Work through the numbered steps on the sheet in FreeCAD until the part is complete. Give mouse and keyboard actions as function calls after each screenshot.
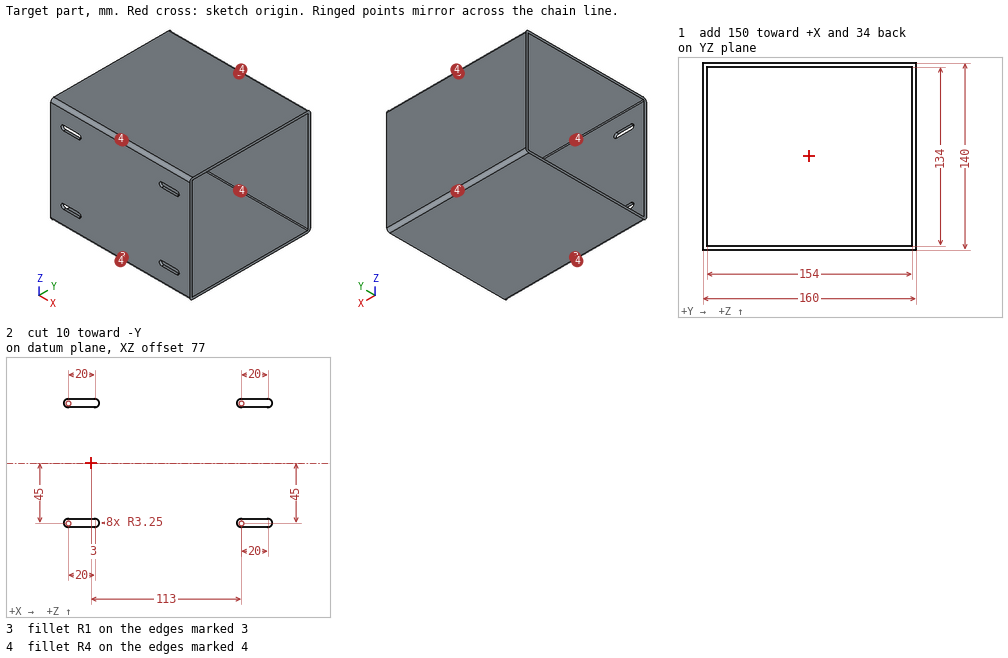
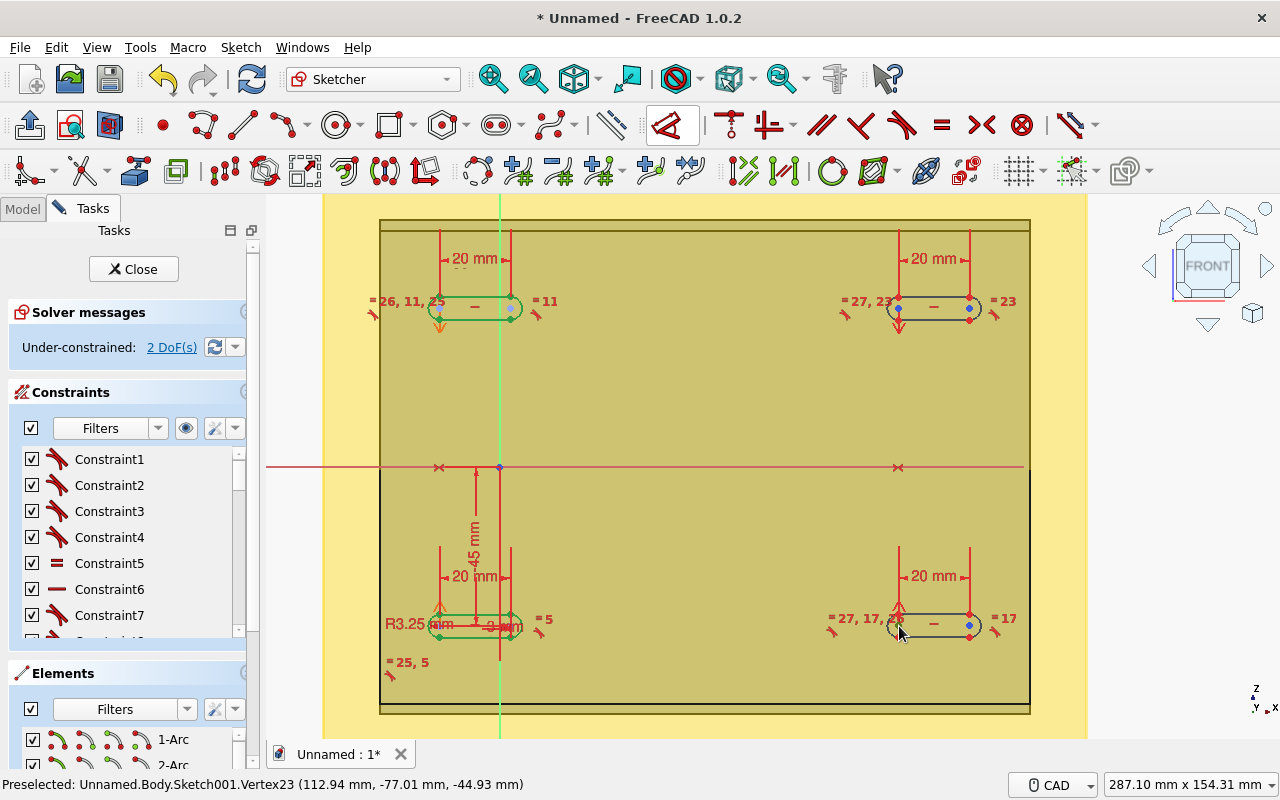
key(i)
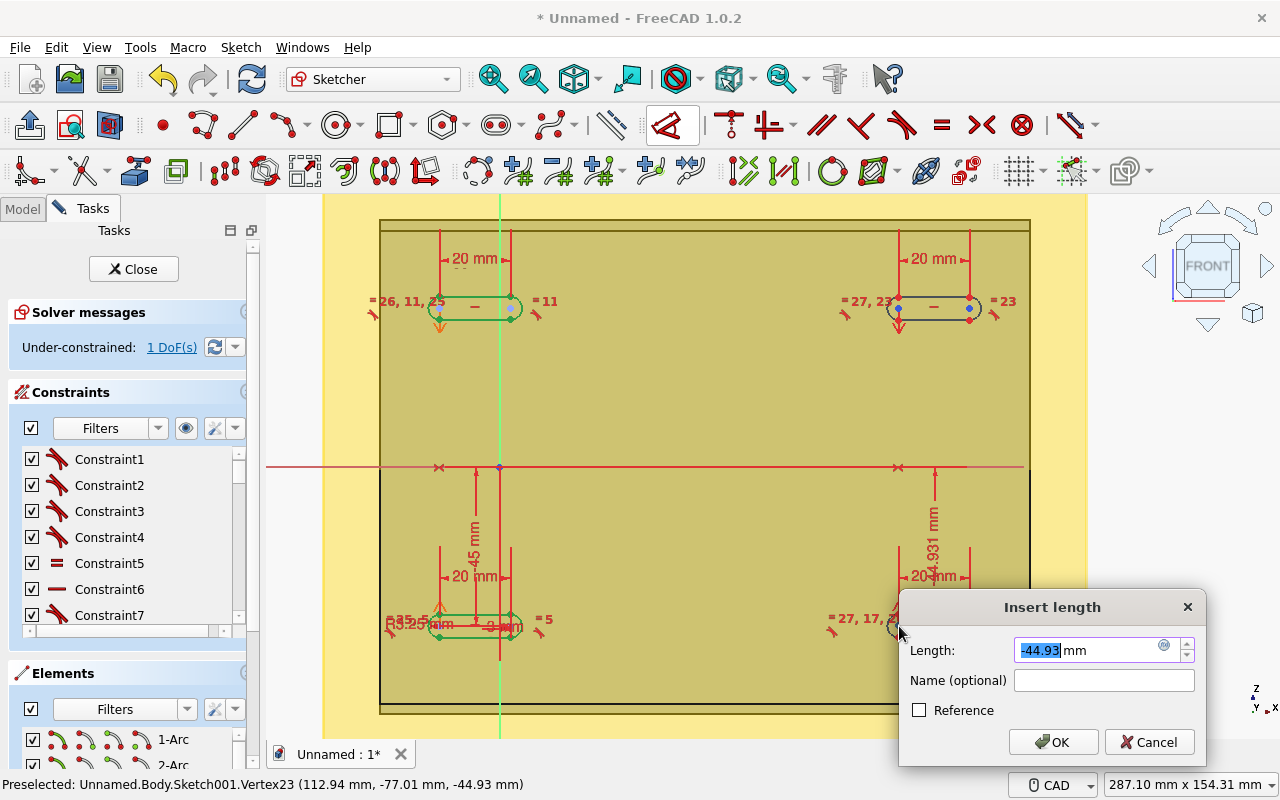
text(-45)
key(Return)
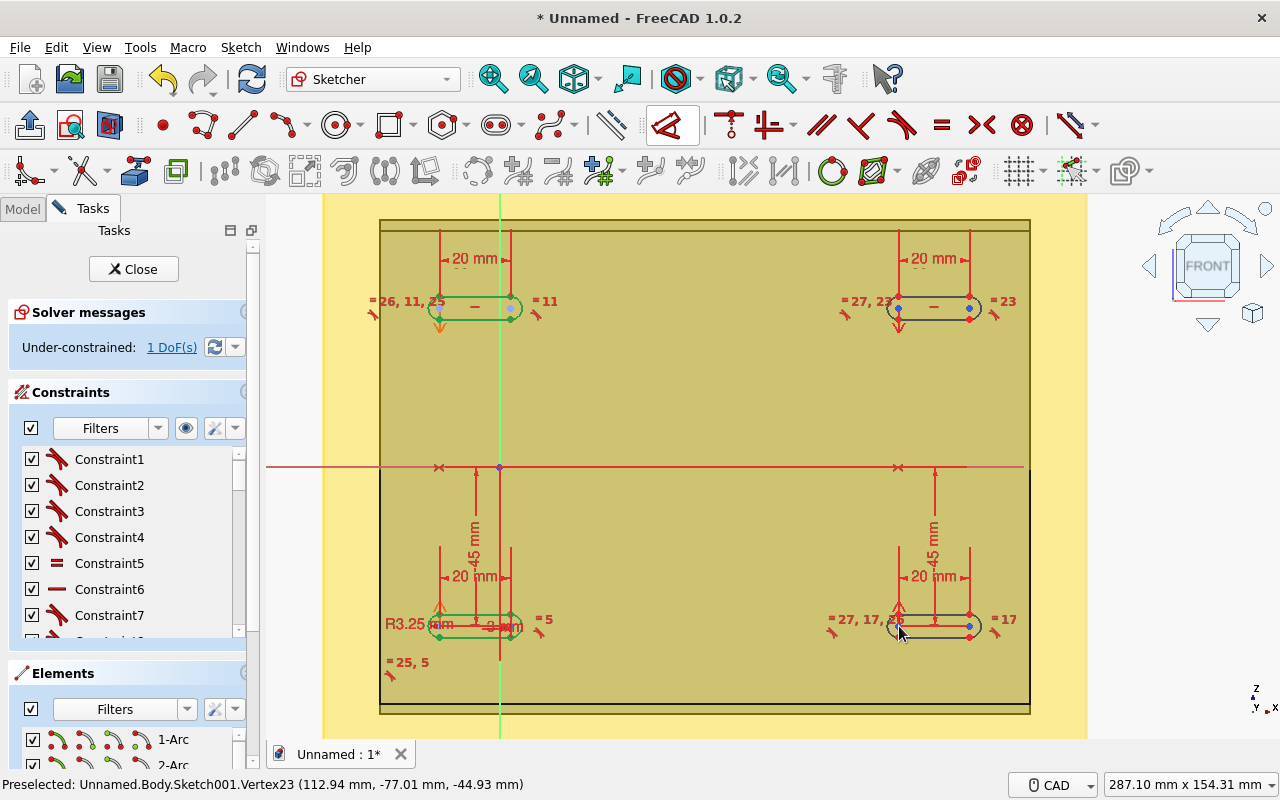
click(899, 615)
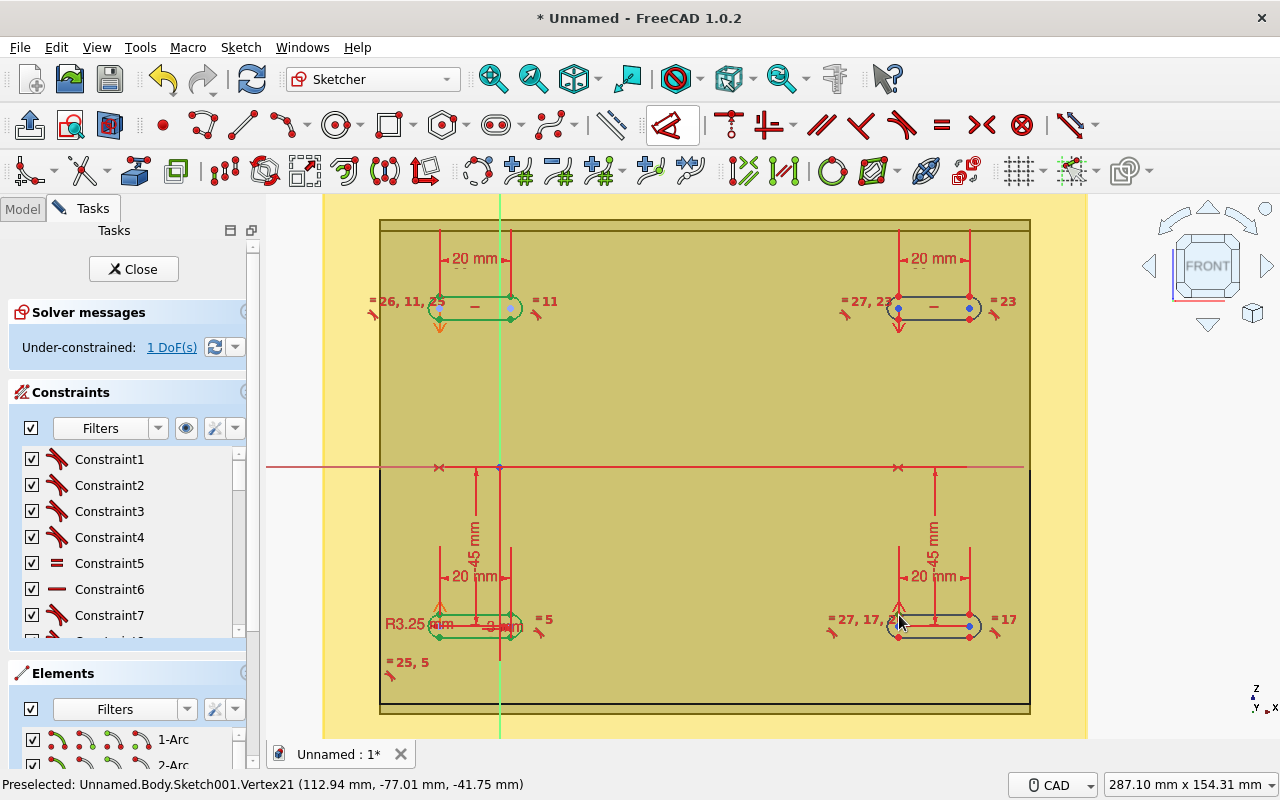
key(l)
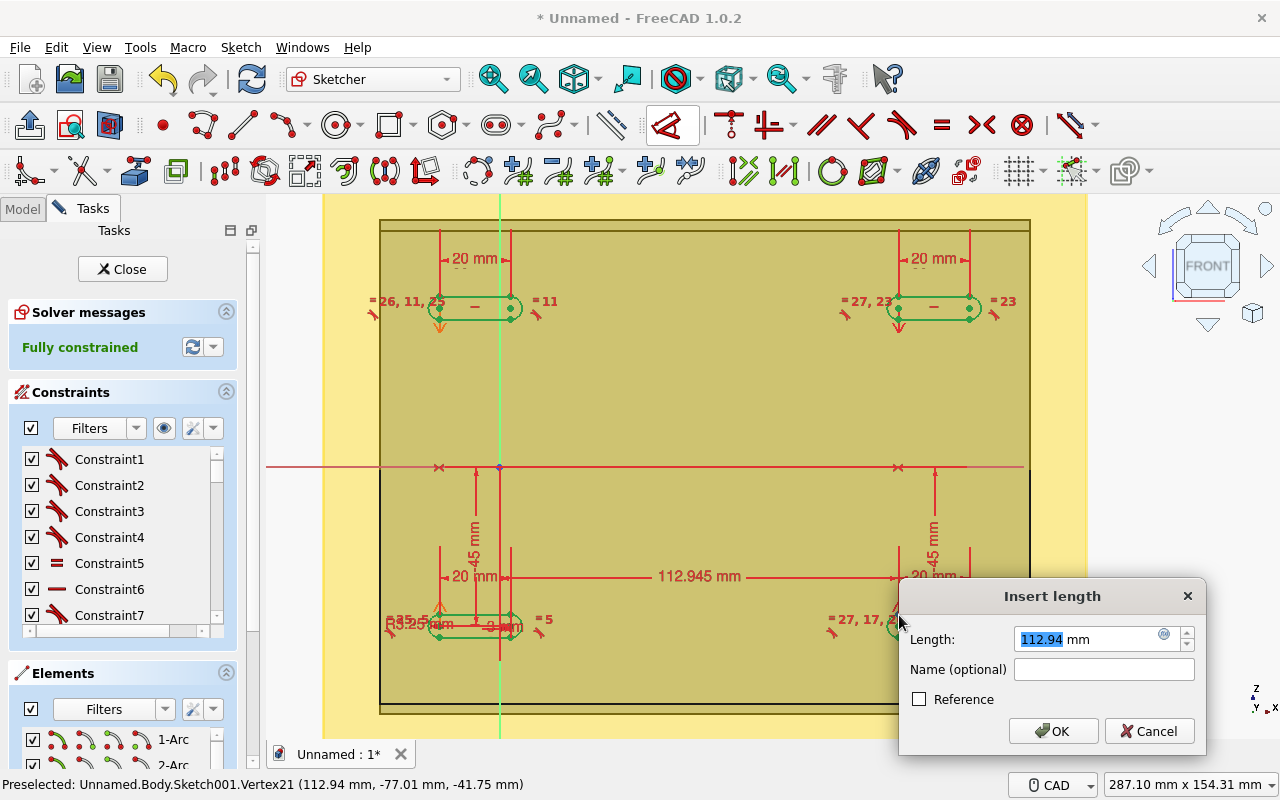
text(113)
key(Return)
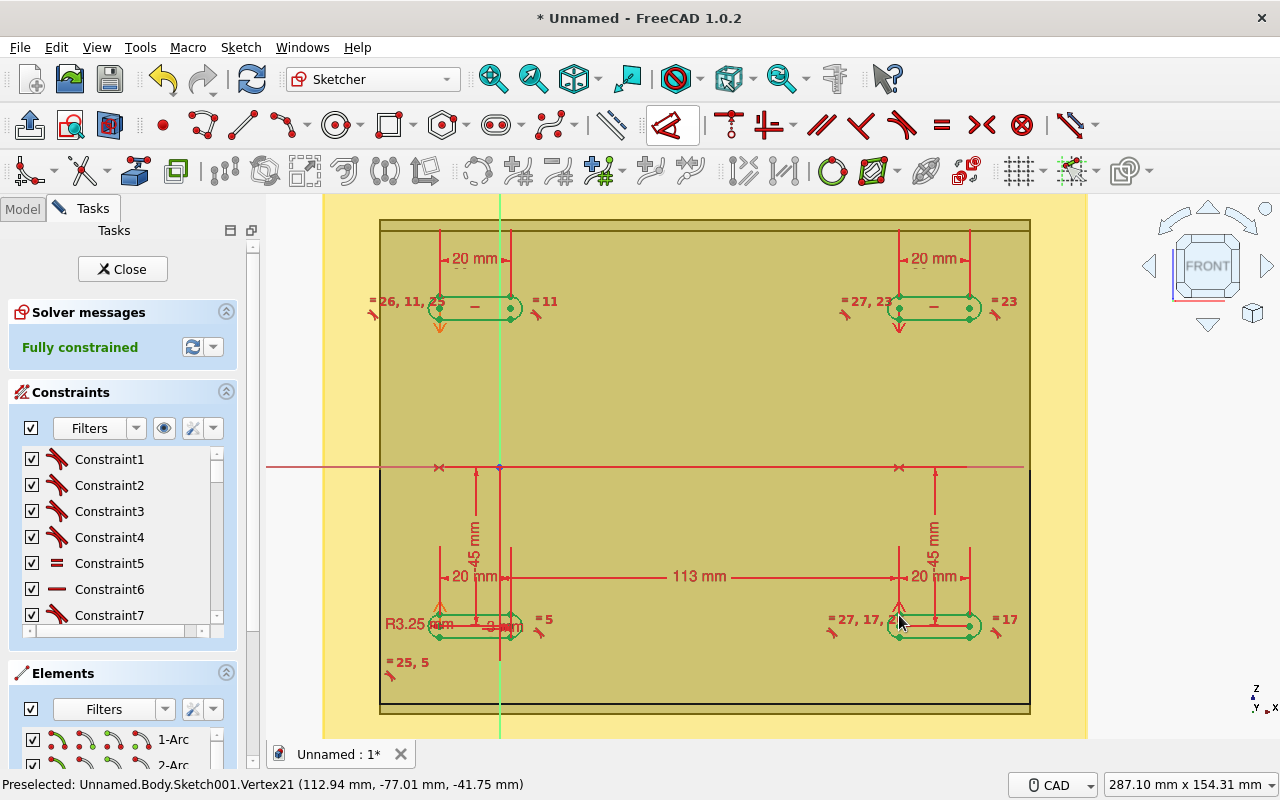
click(123, 269)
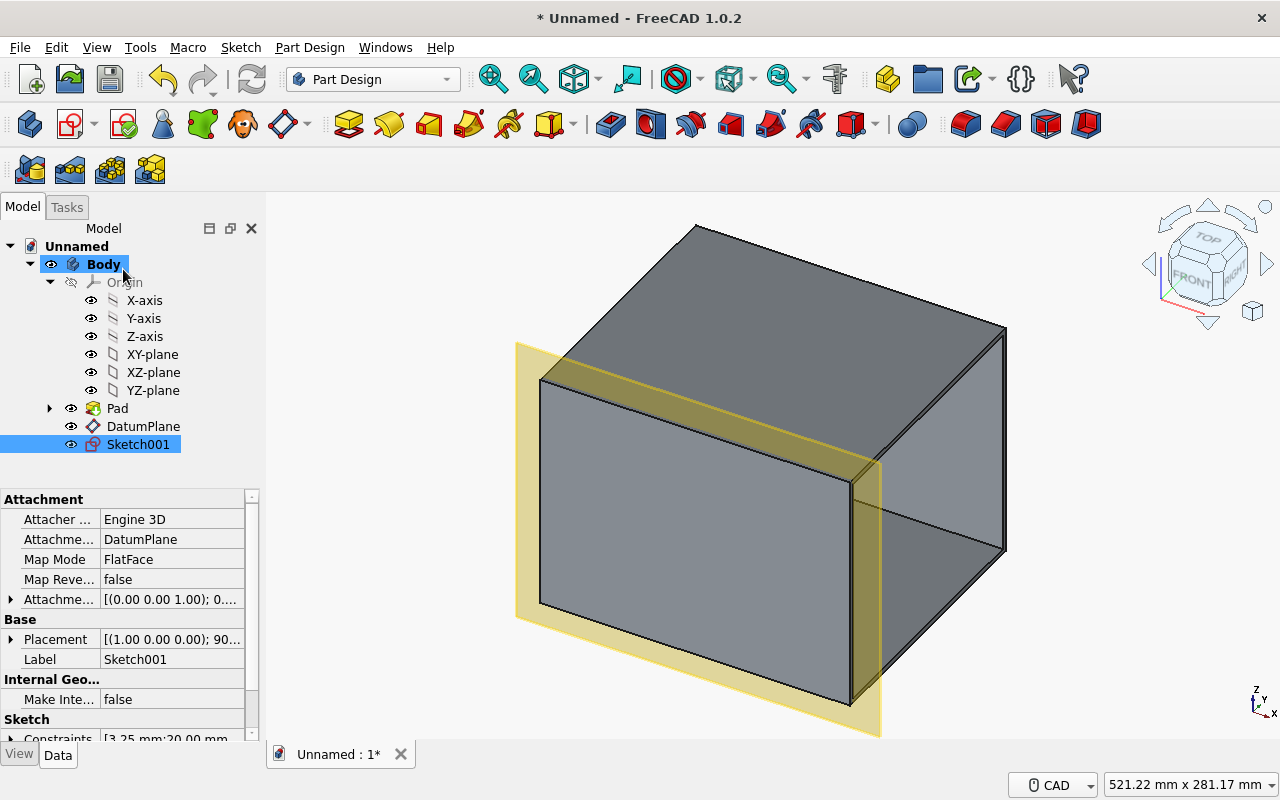
click(612, 124)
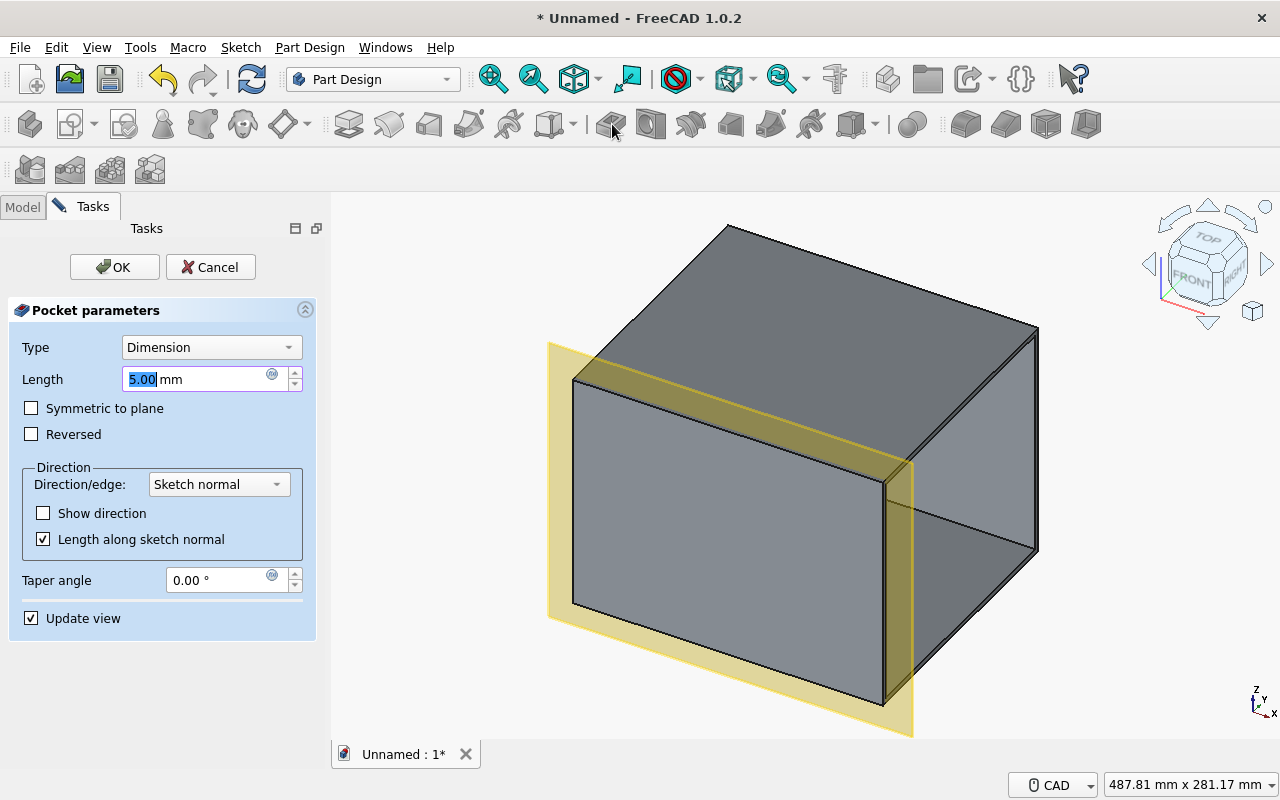
text(10)
key(Tab)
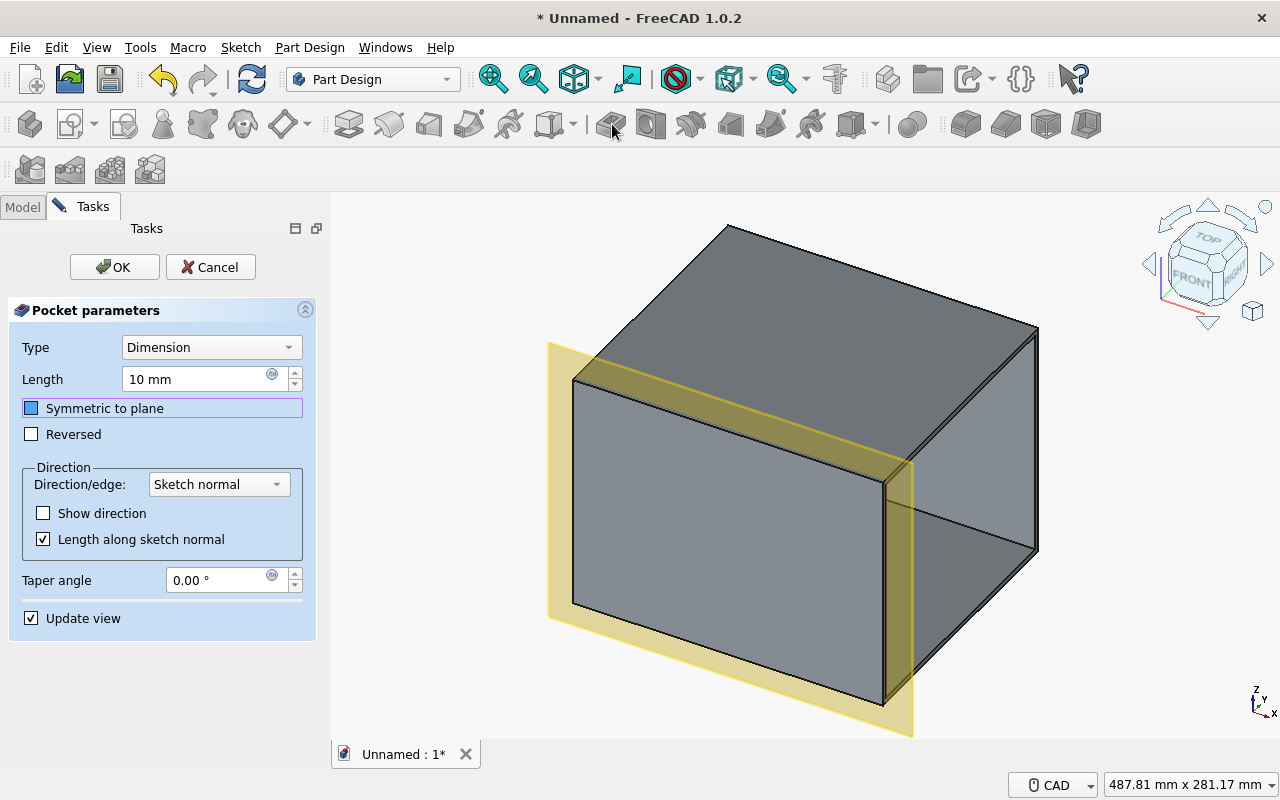
click(30, 434)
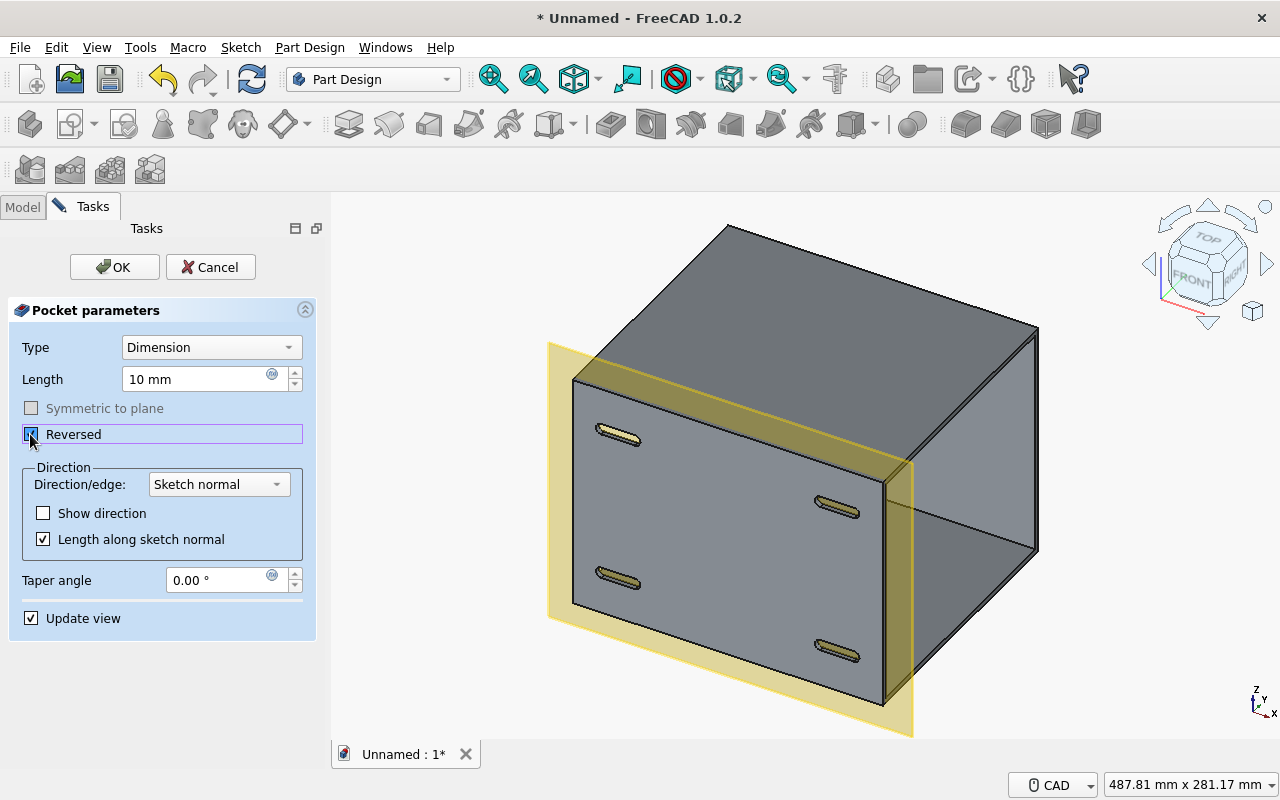
click(115, 267)